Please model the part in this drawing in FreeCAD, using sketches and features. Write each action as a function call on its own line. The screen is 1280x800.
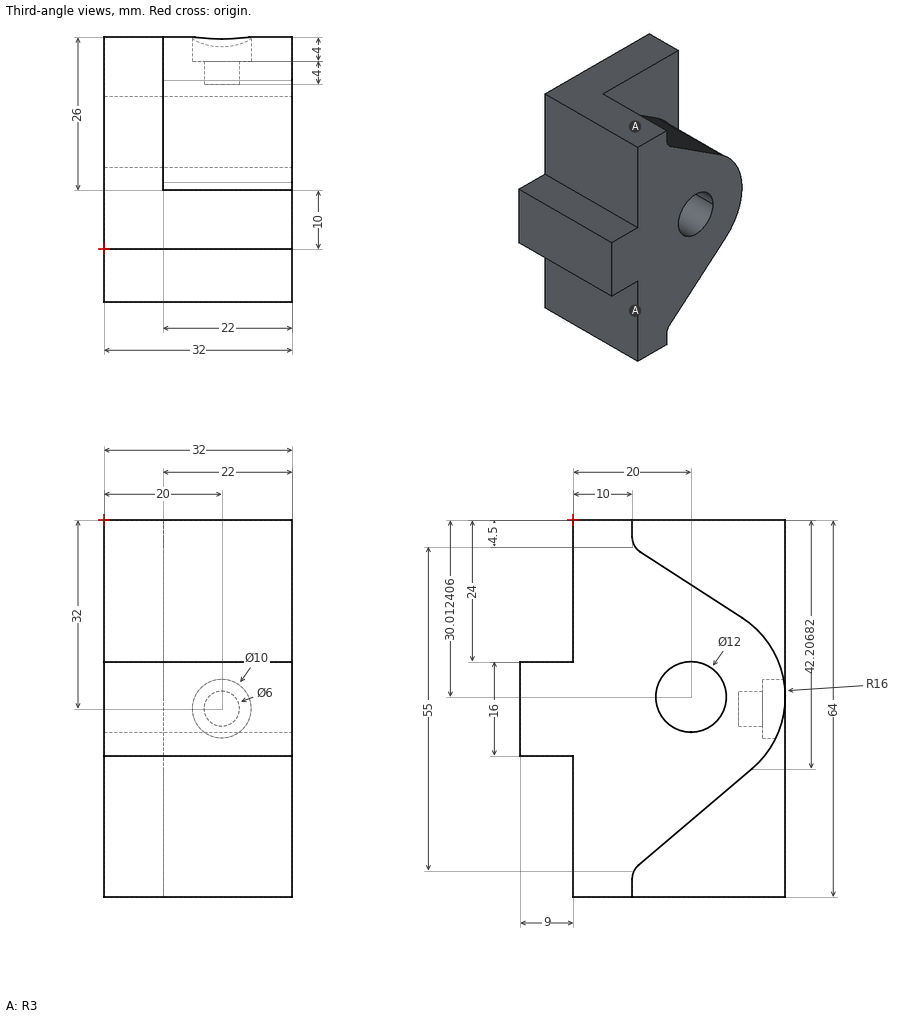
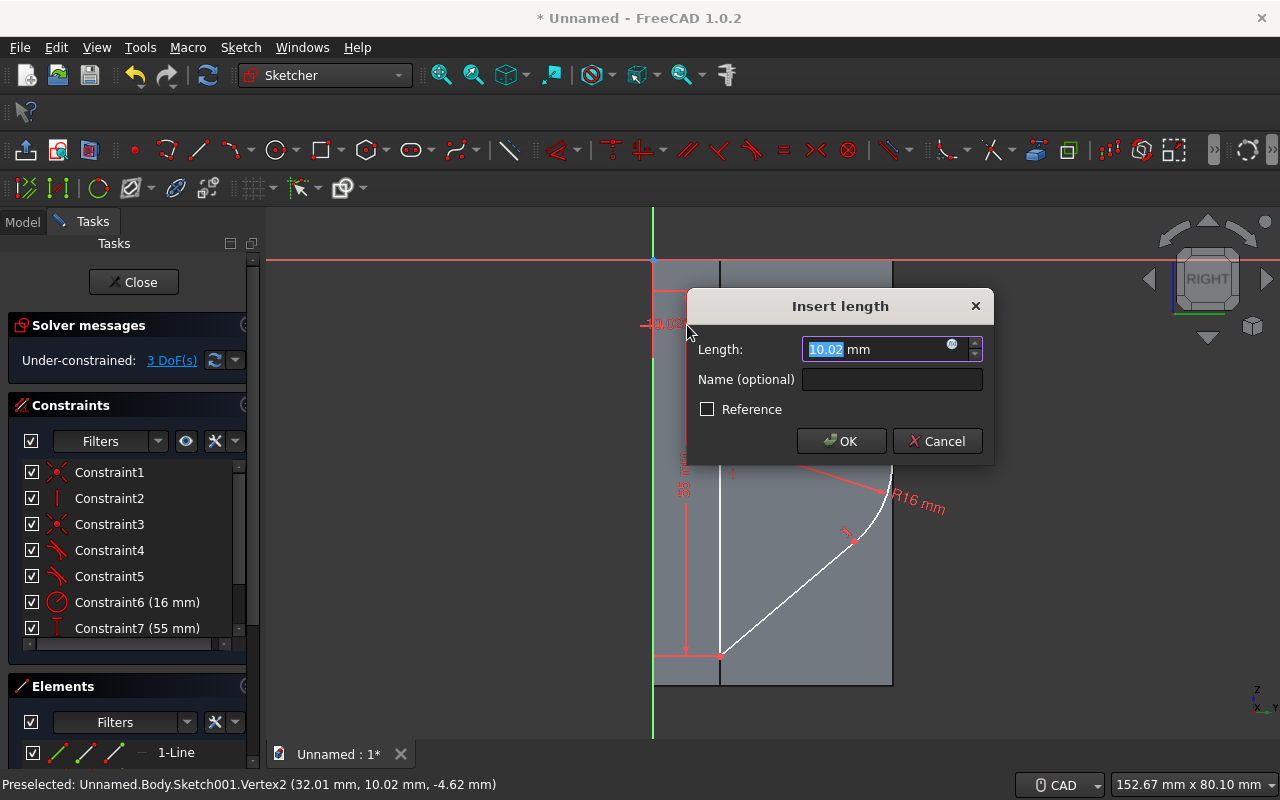
text(10)
key(Return)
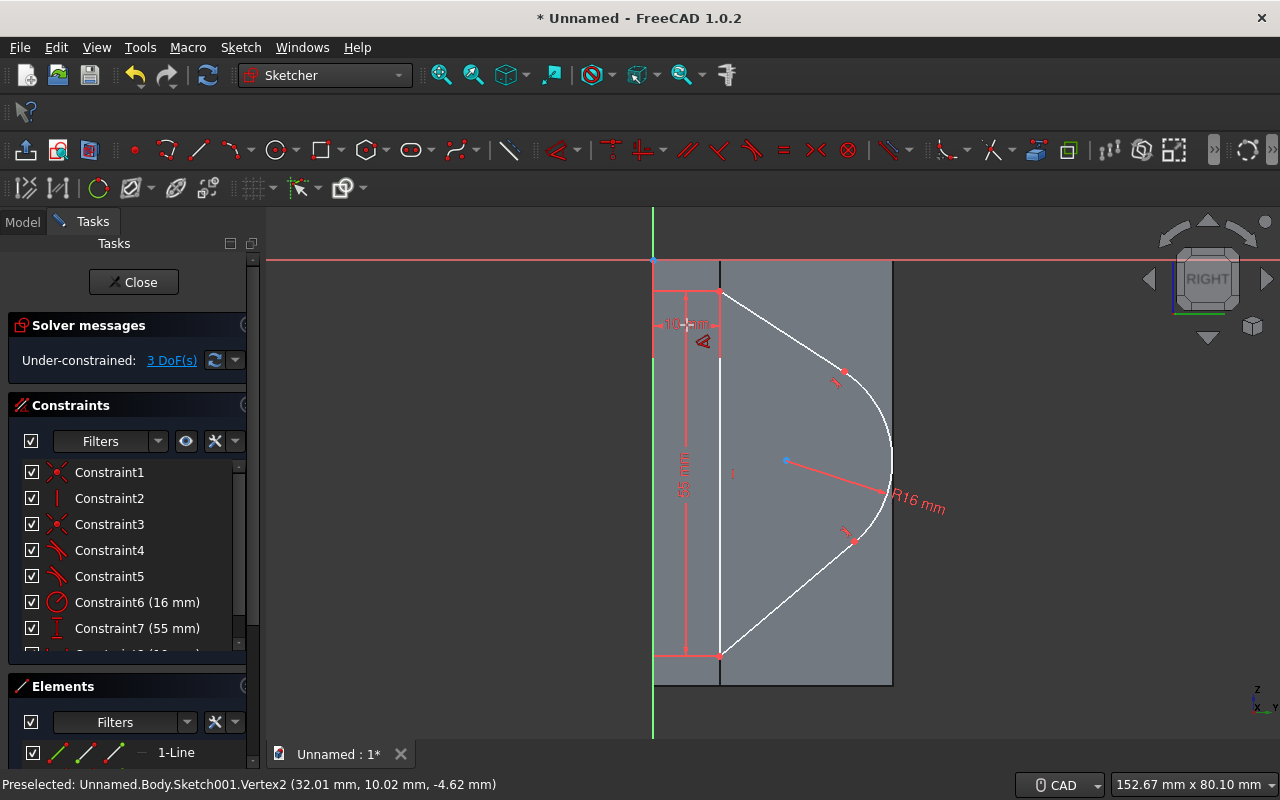
click(786, 461)
click(689, 495)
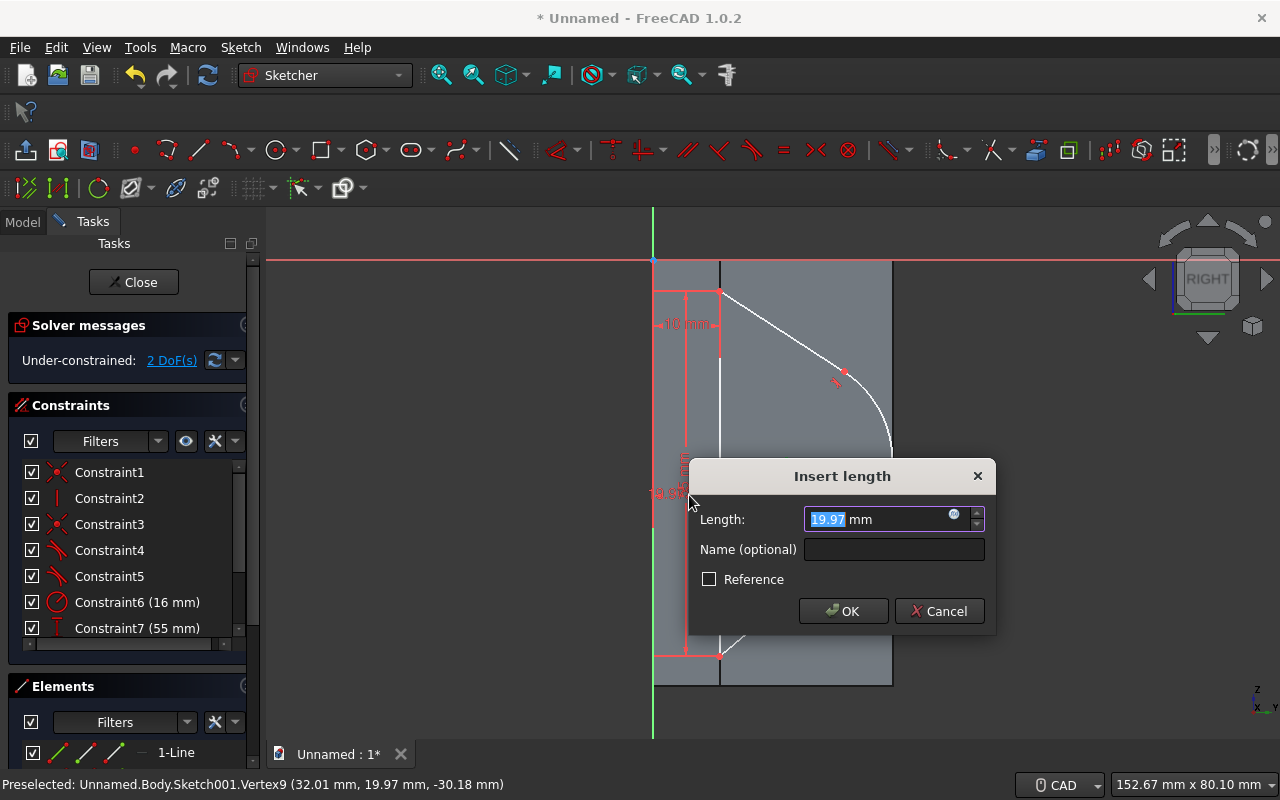
text(20)
key(Return)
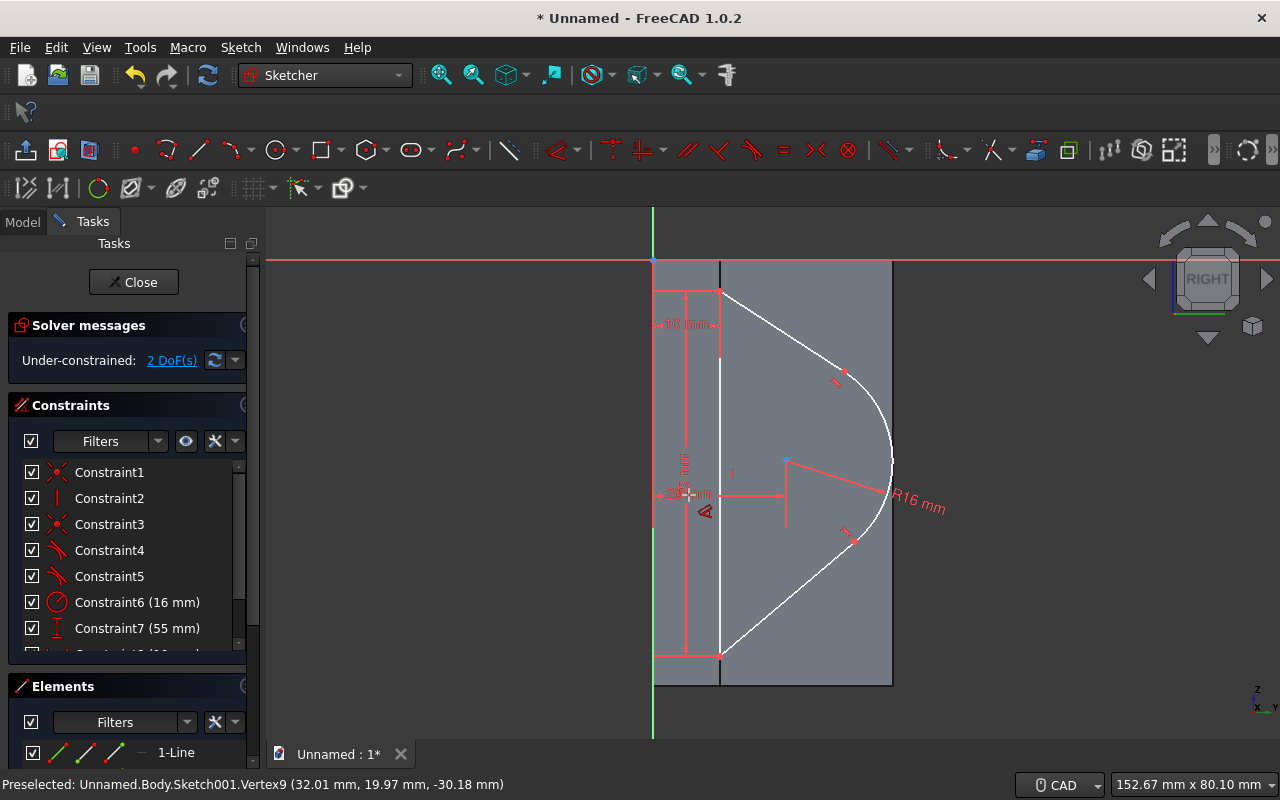
scroll(720, 291, up, 2)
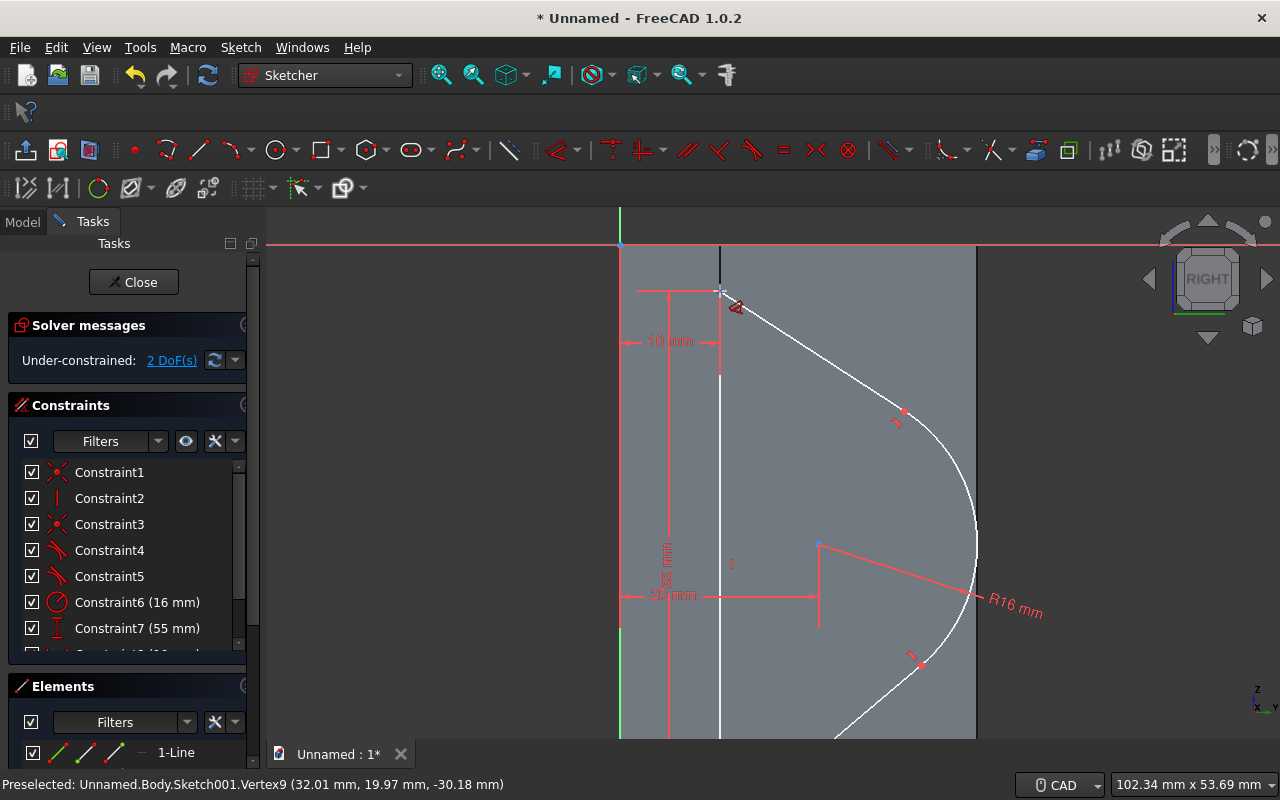
click(720, 291)
click(586, 268)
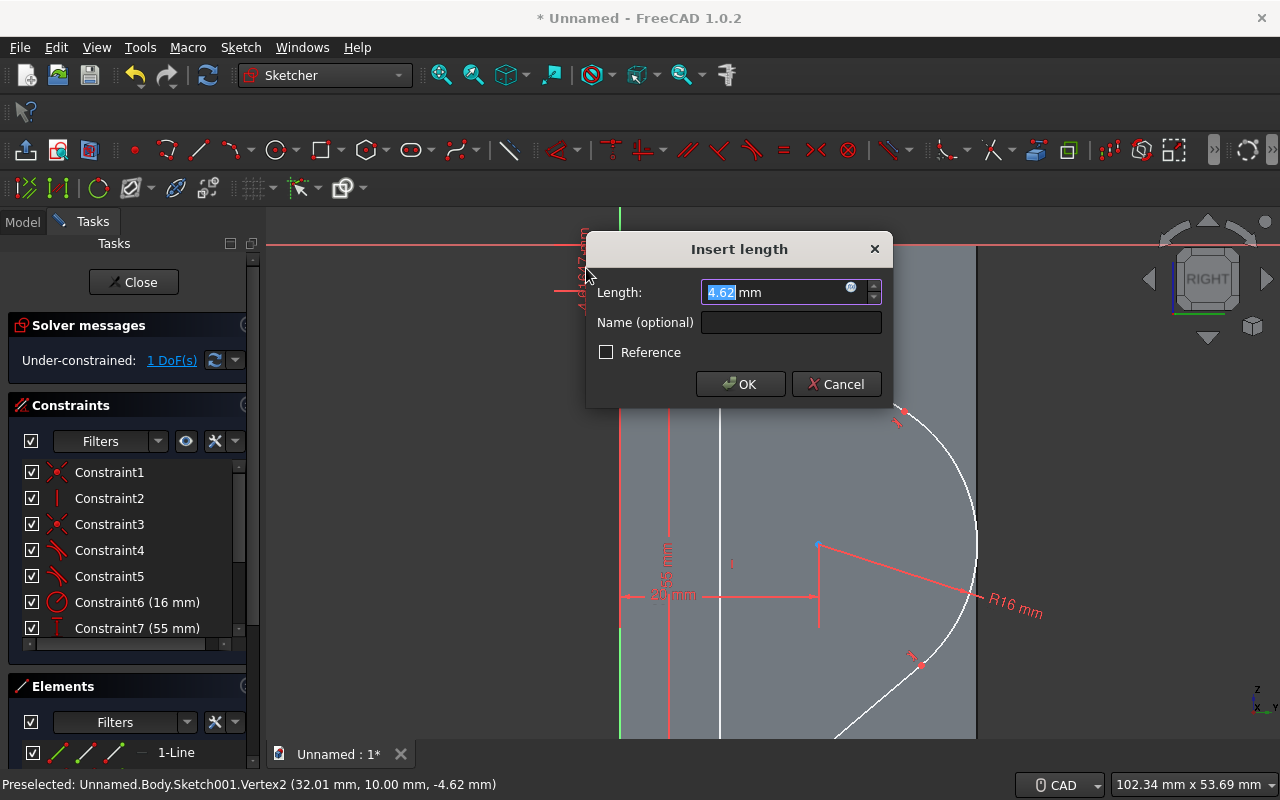
text(4.5)
key(Return)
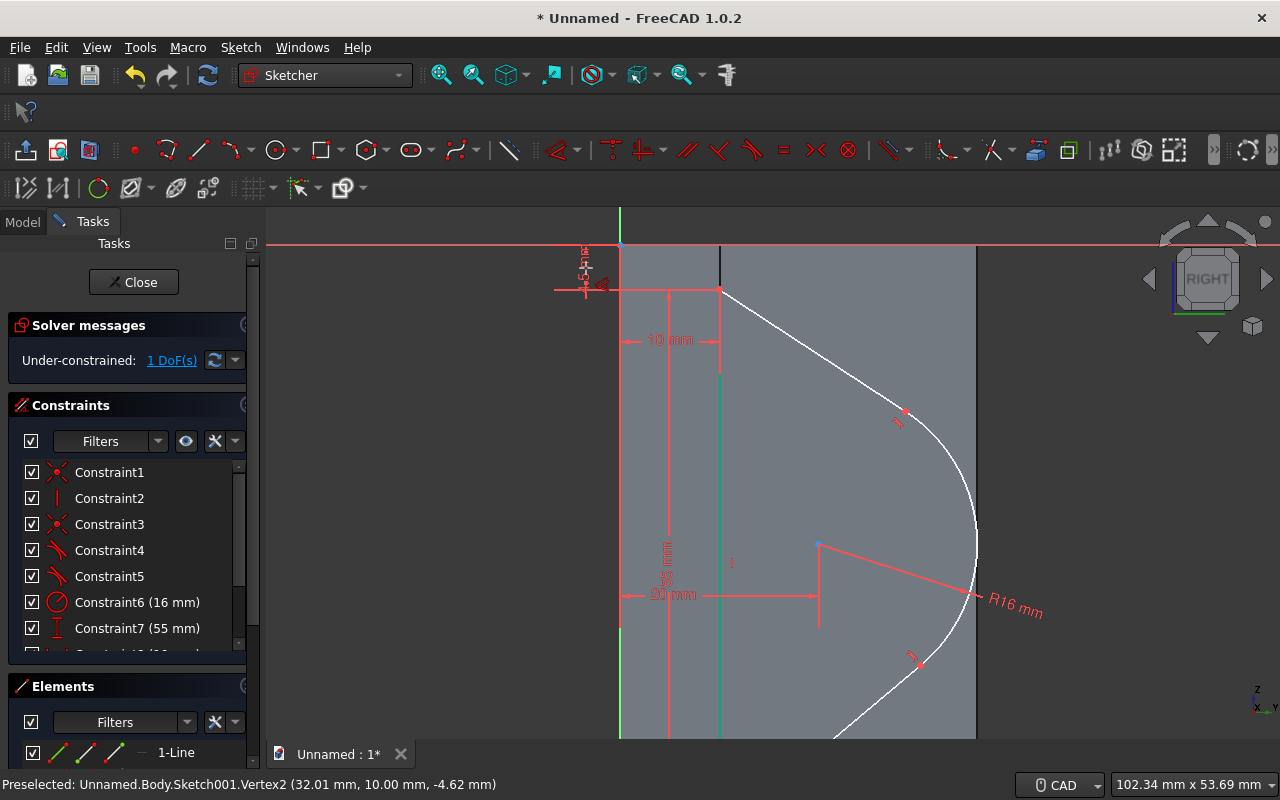
click(921, 665)
click(586, 455)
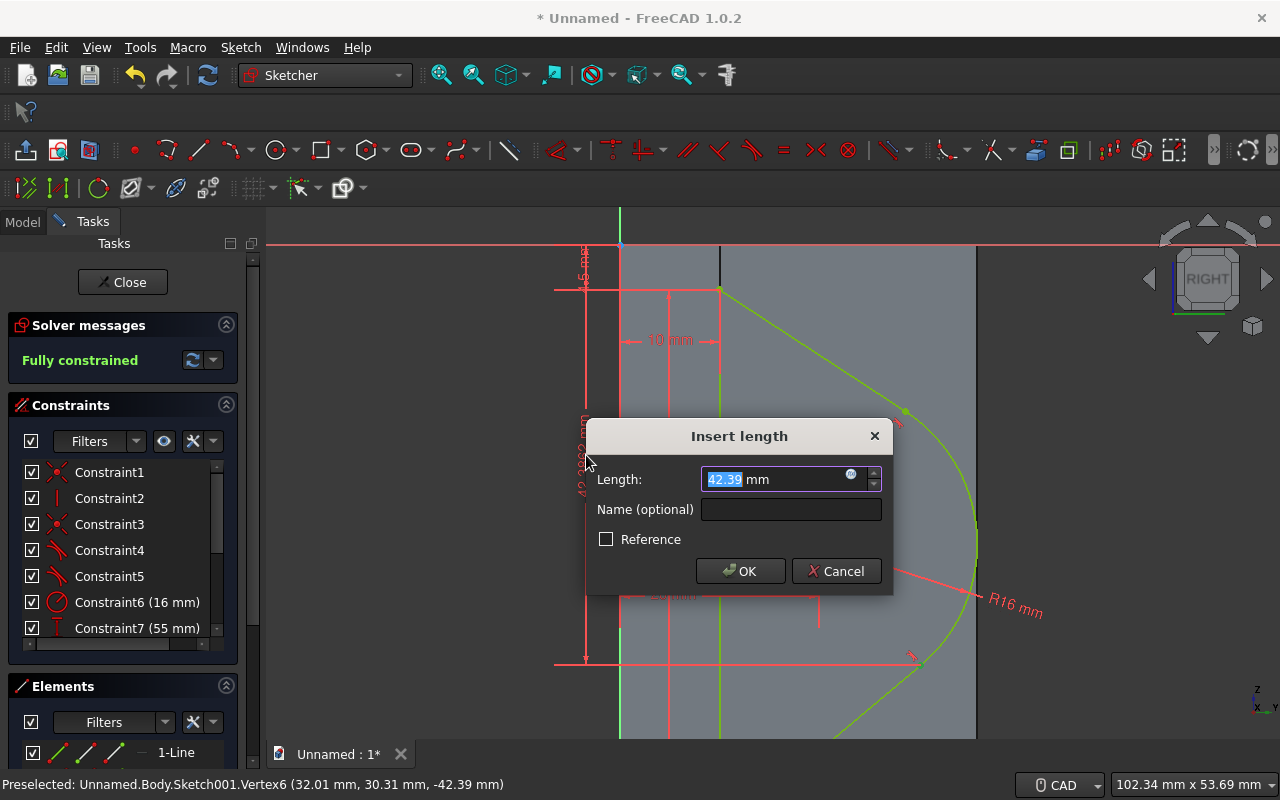
text(42.20682)
key(Return)
key(Escape)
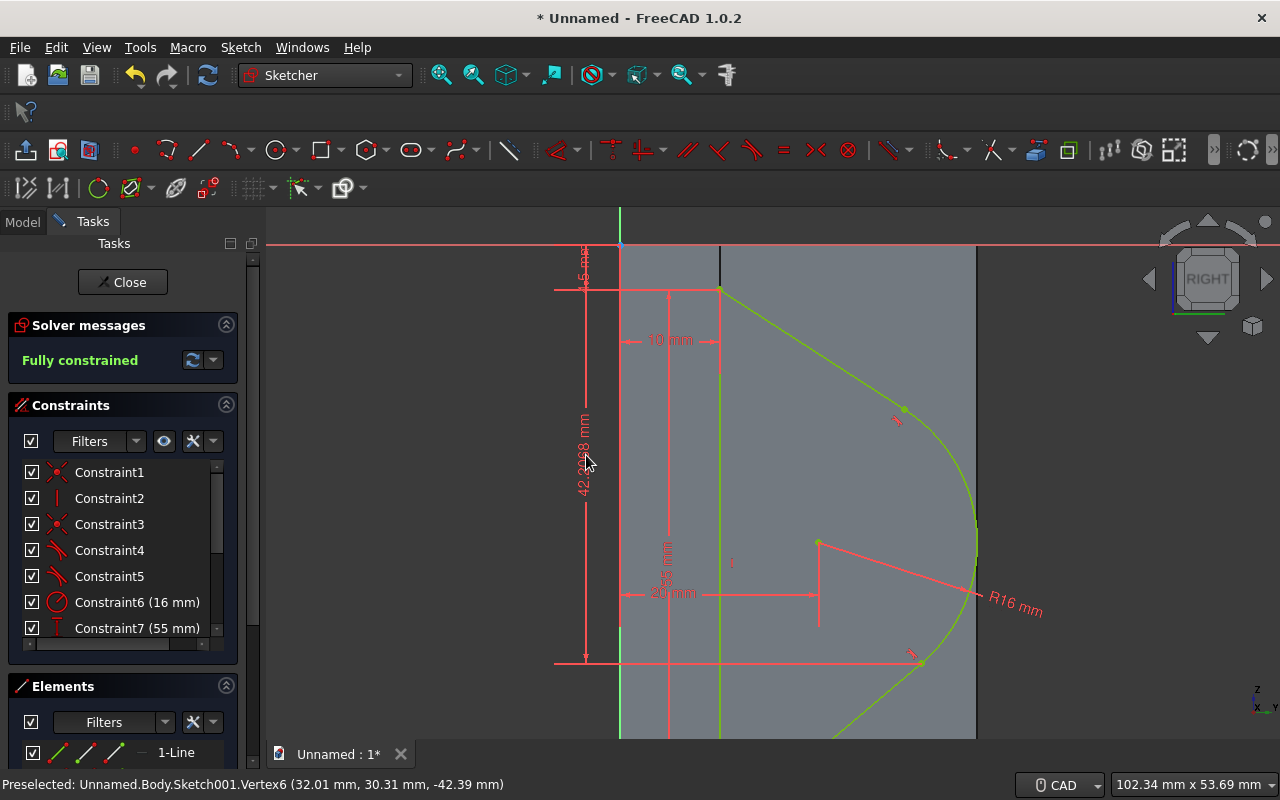
click(123, 282)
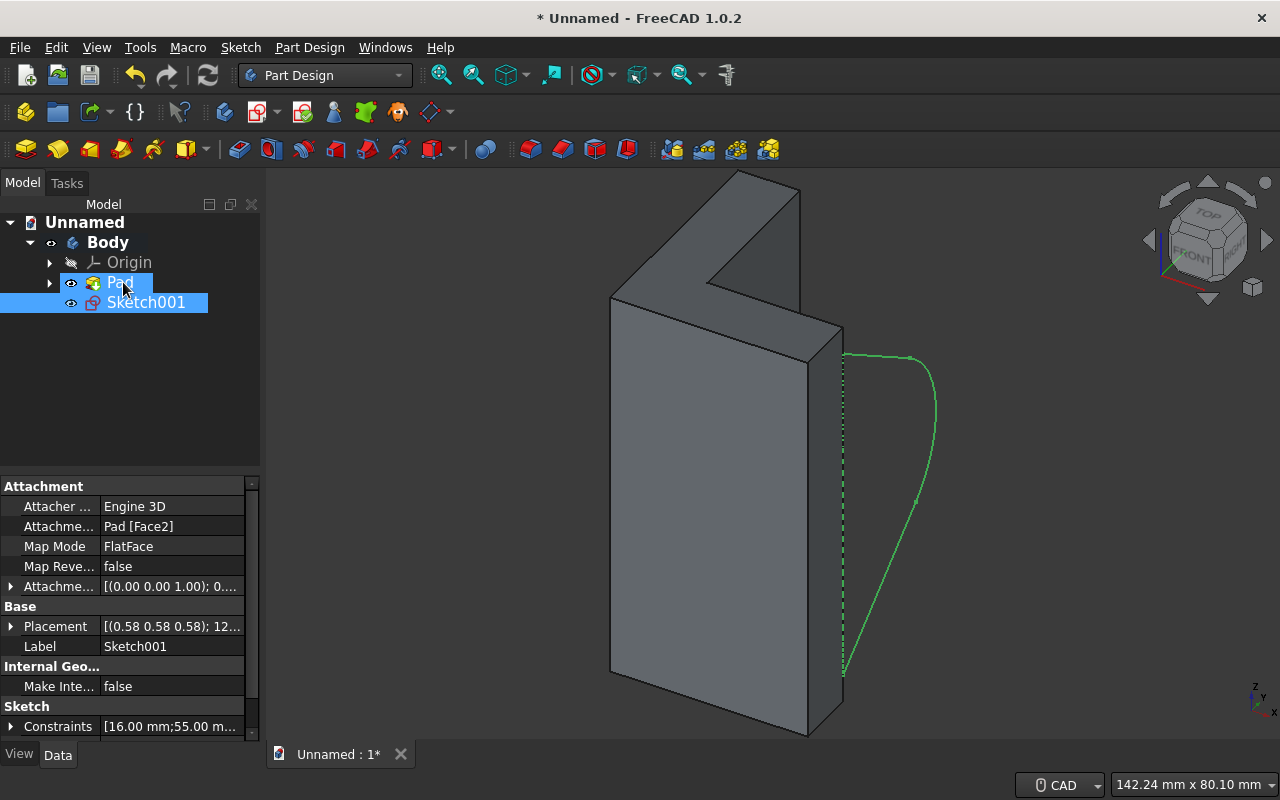
click(26, 150)